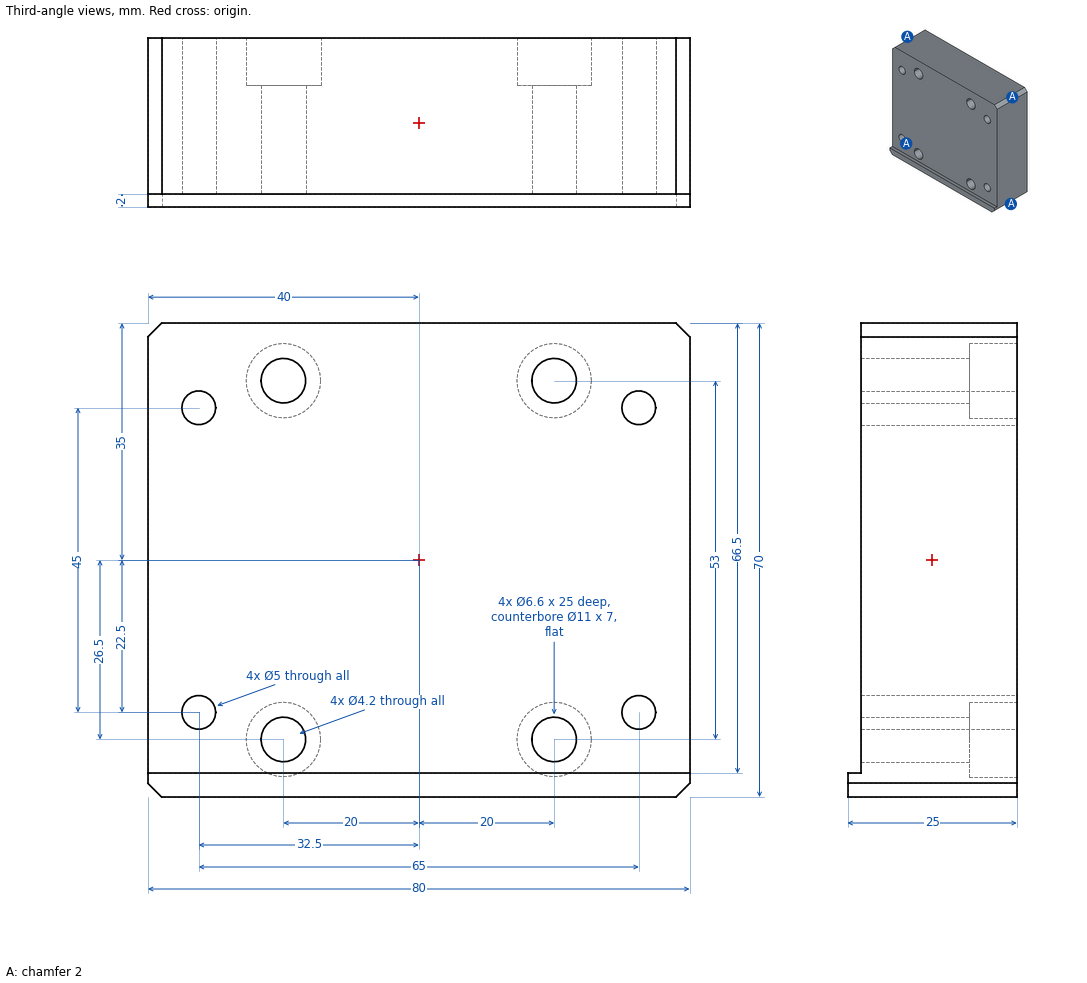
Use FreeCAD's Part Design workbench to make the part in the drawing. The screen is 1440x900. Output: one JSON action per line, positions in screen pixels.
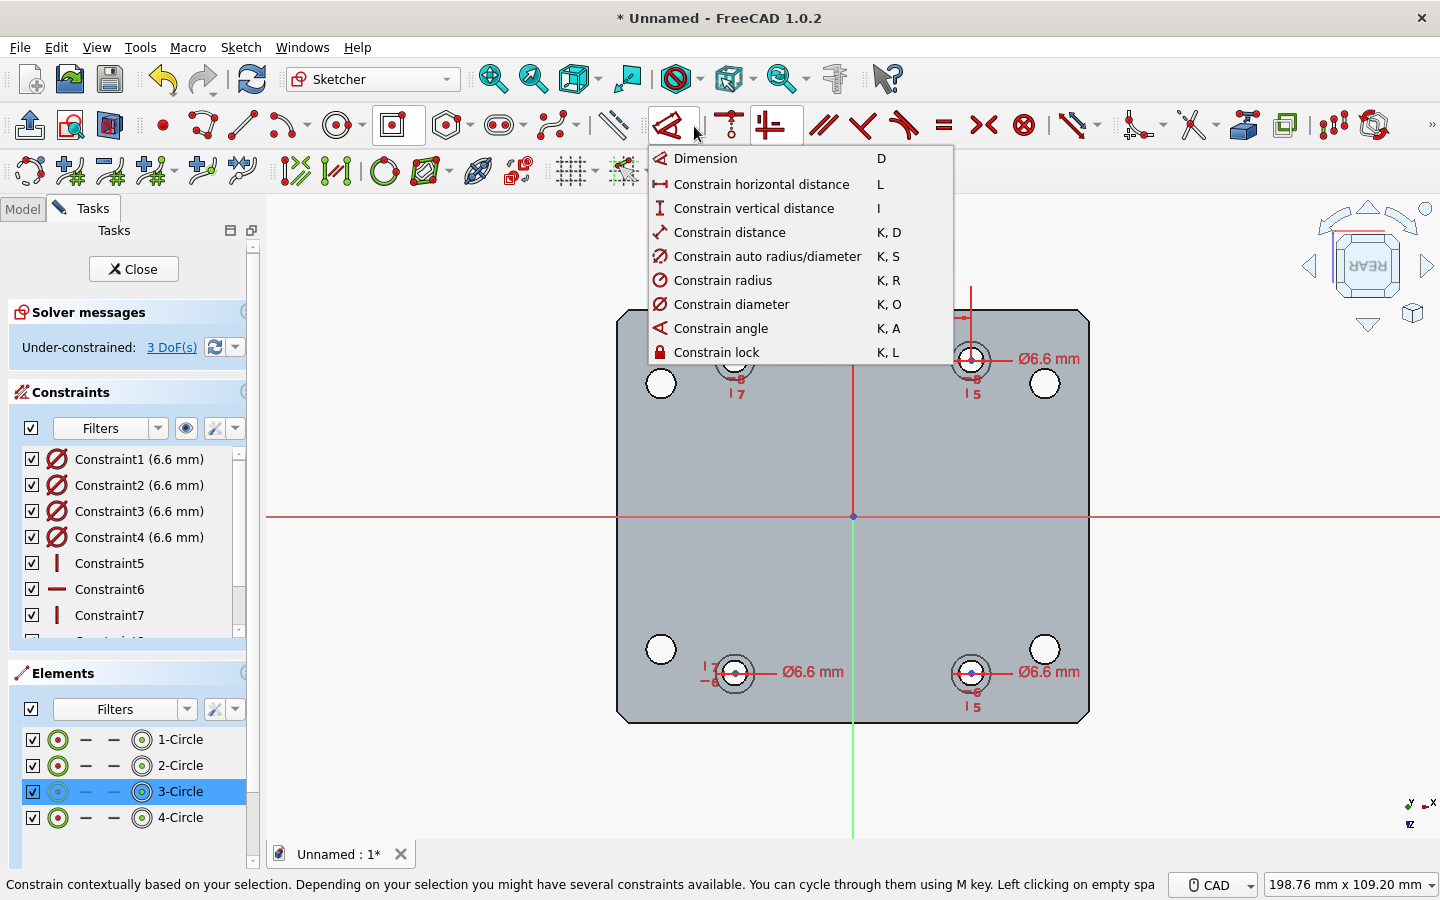
{"action": "left_click", "coordinate": [801, 184]}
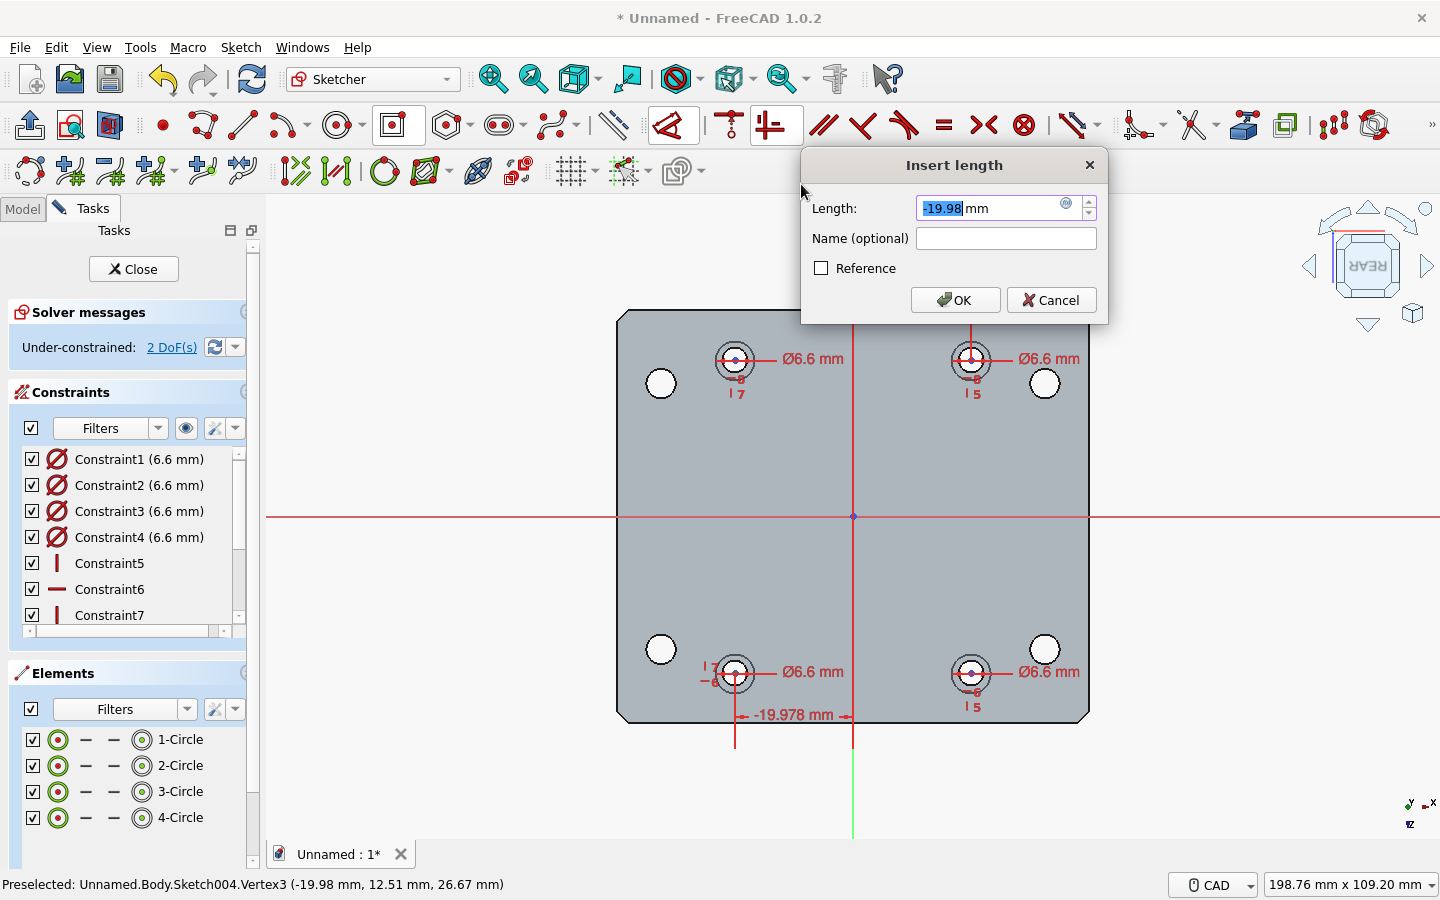
{"action": "type", "text": "-20"}
{"action": "key", "text": "Return"}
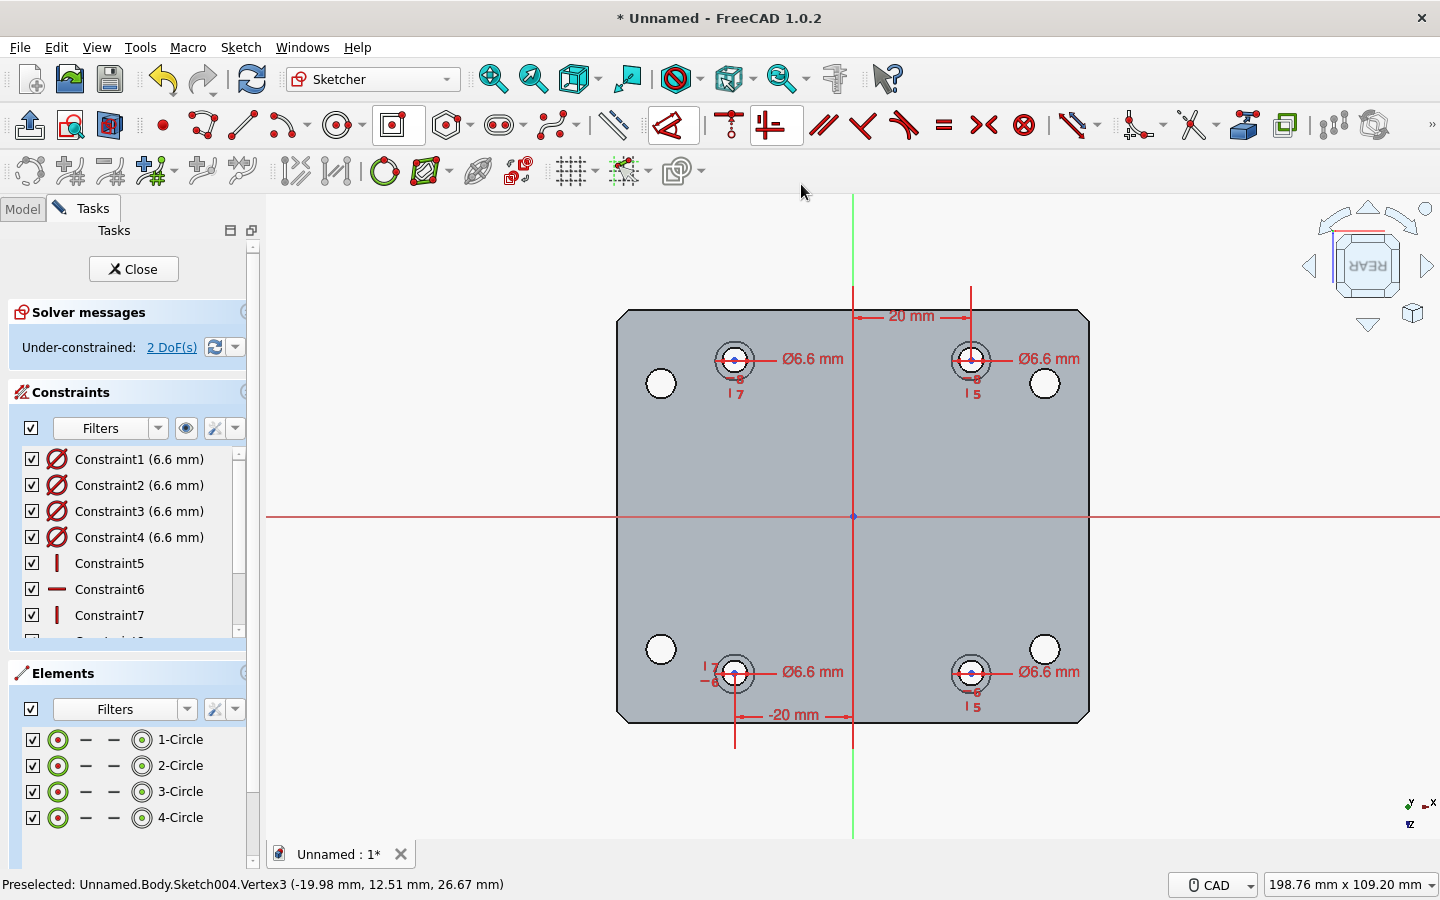
{"action": "left_click", "coordinate": [971, 361]}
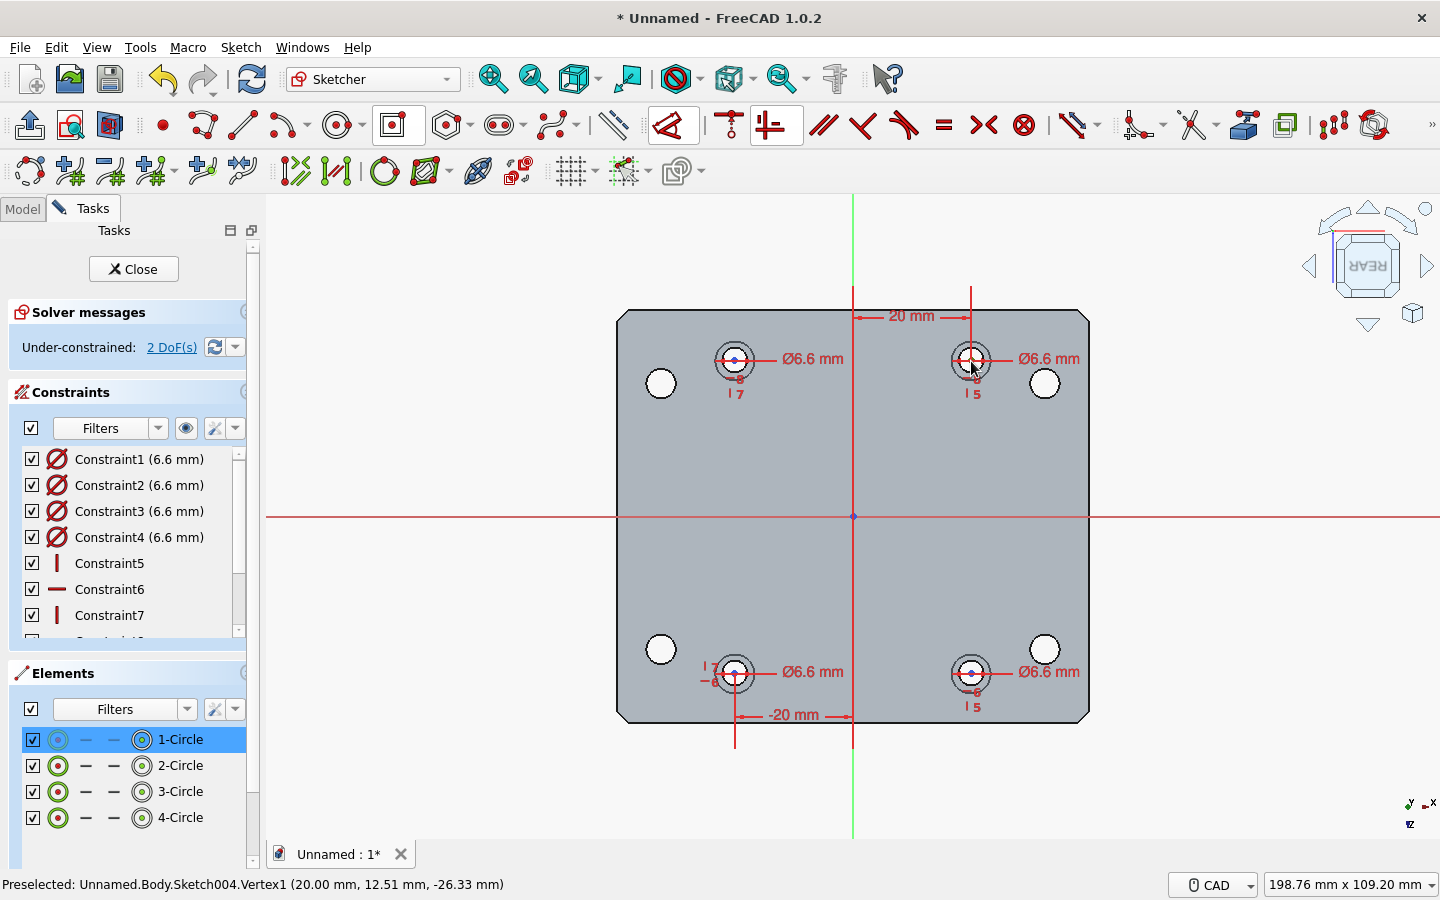
{"action": "left_click", "coordinate": [971, 674]}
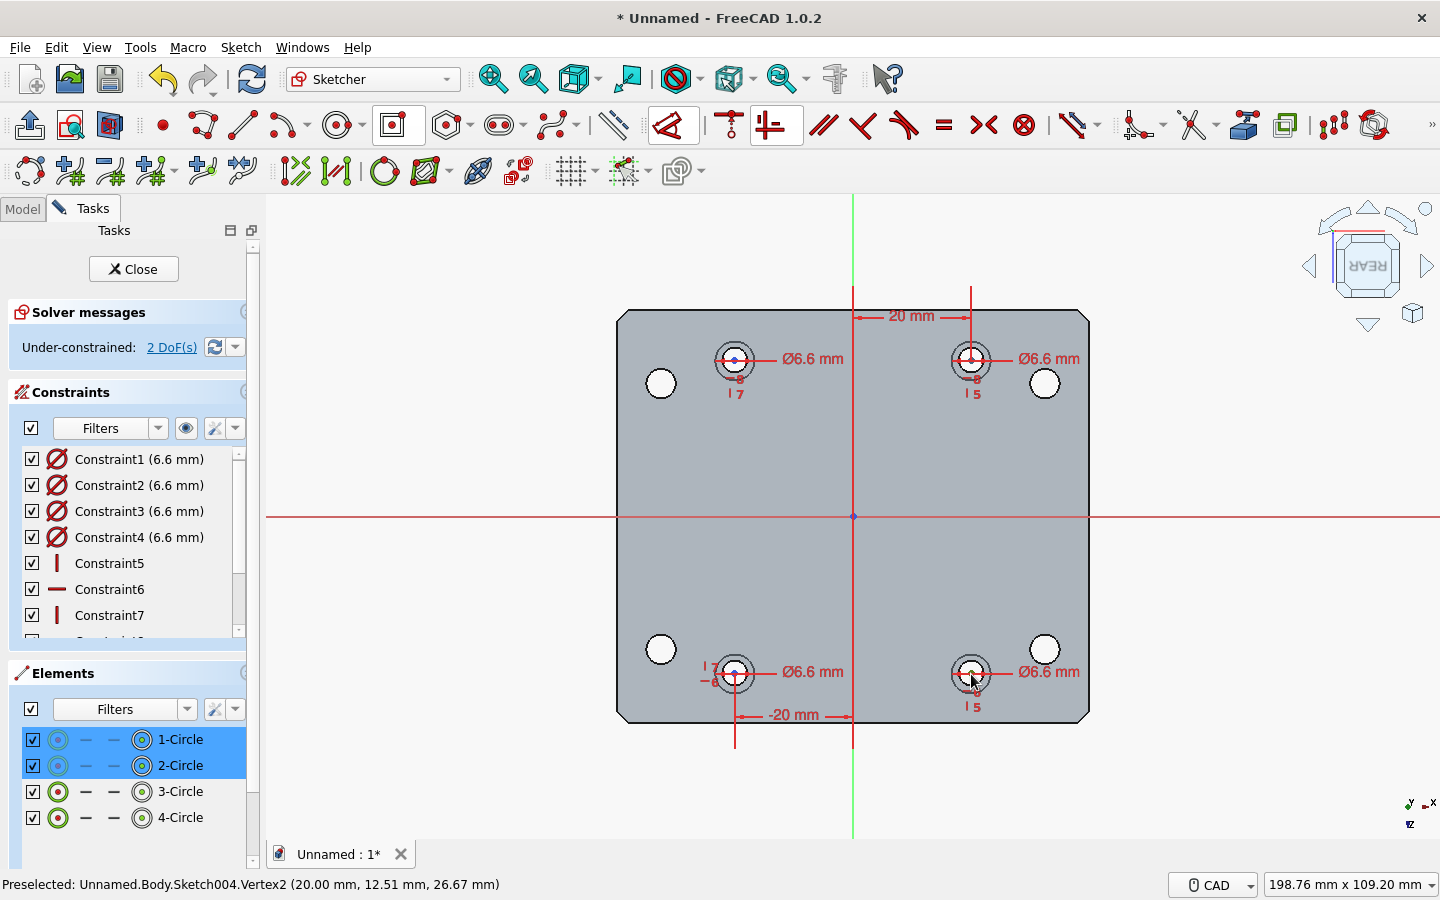
{"action": "left_click", "coordinate": [694, 126]}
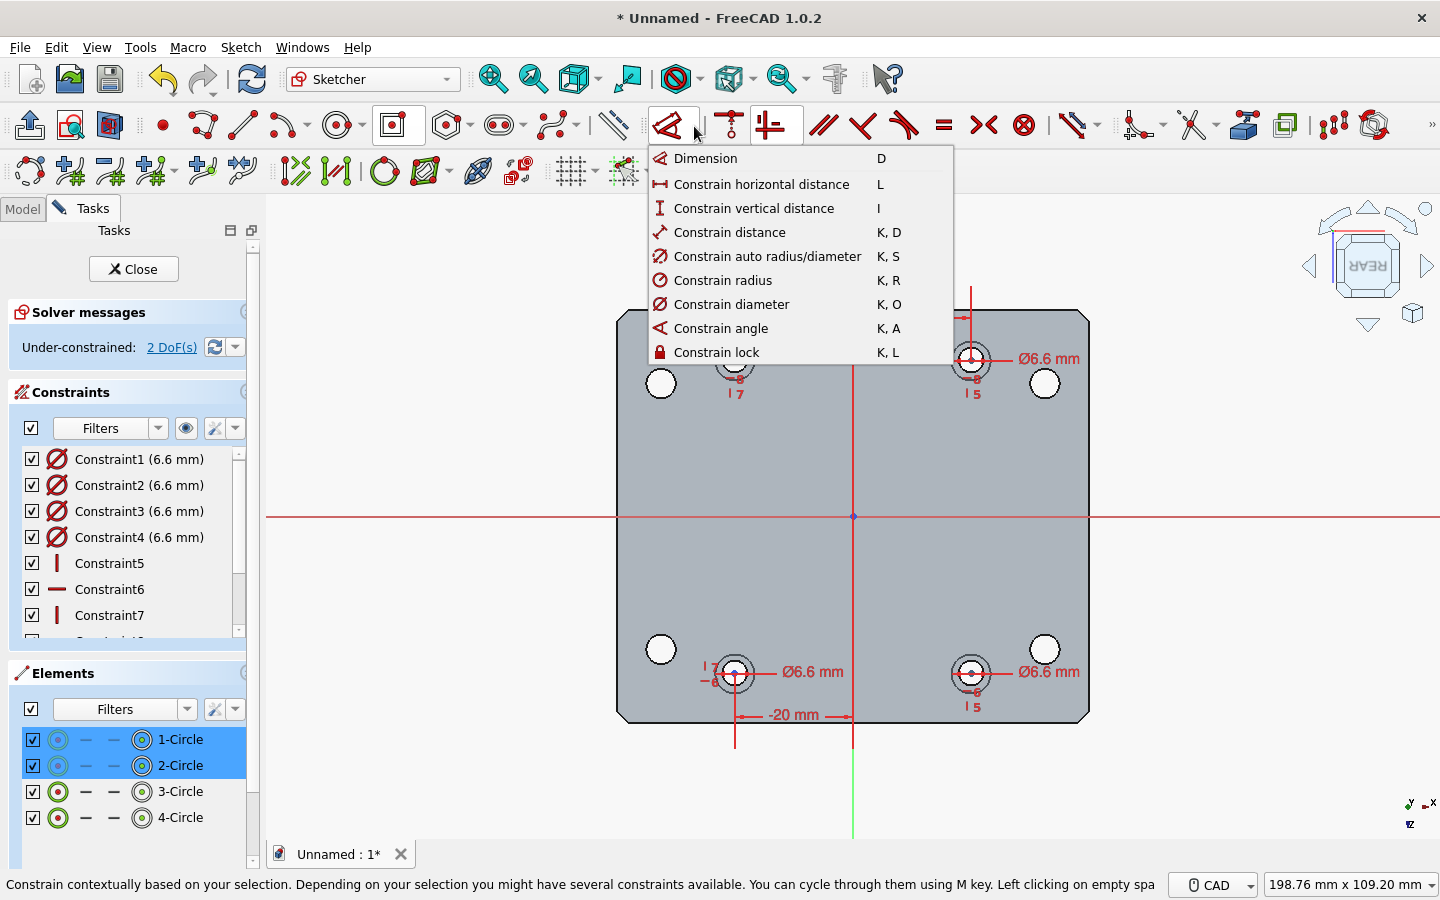
{"action": "left_click", "coordinate": [801, 208]}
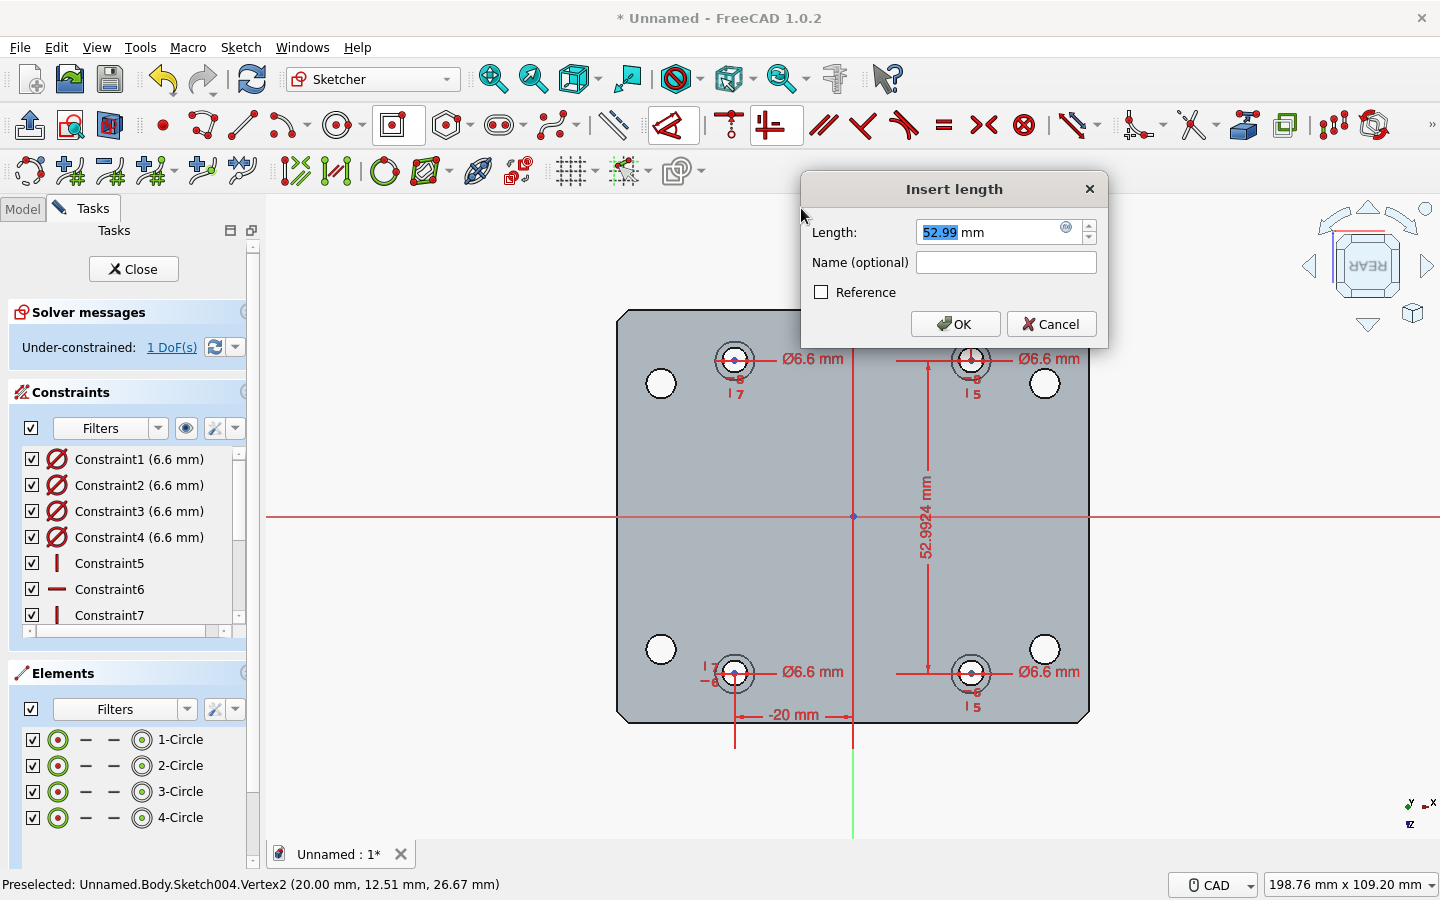
{"action": "type", "text": "53"}
{"action": "key", "text": "Return"}